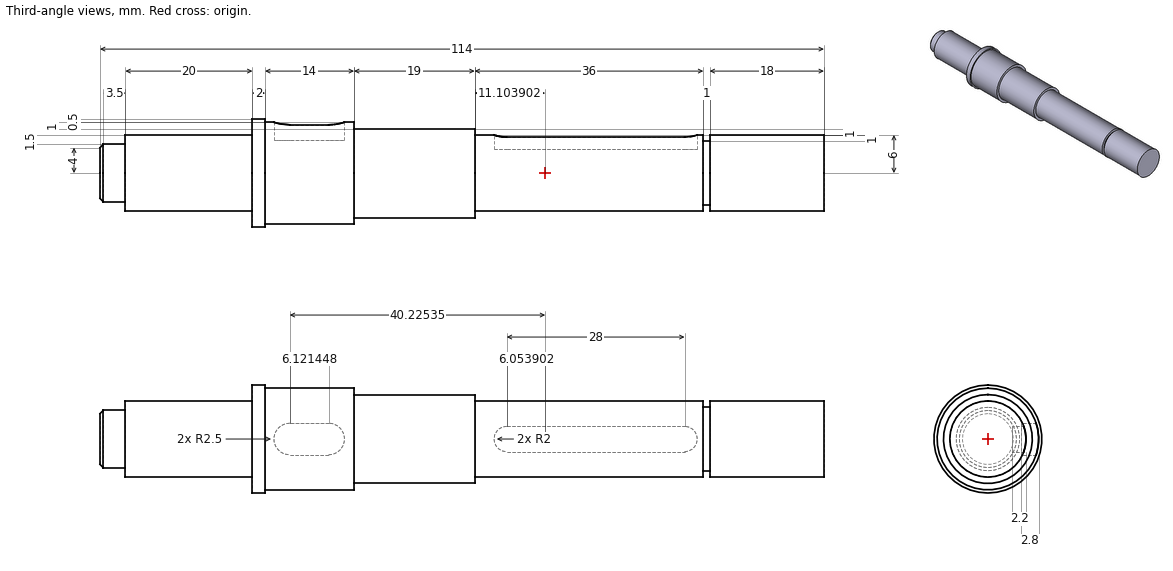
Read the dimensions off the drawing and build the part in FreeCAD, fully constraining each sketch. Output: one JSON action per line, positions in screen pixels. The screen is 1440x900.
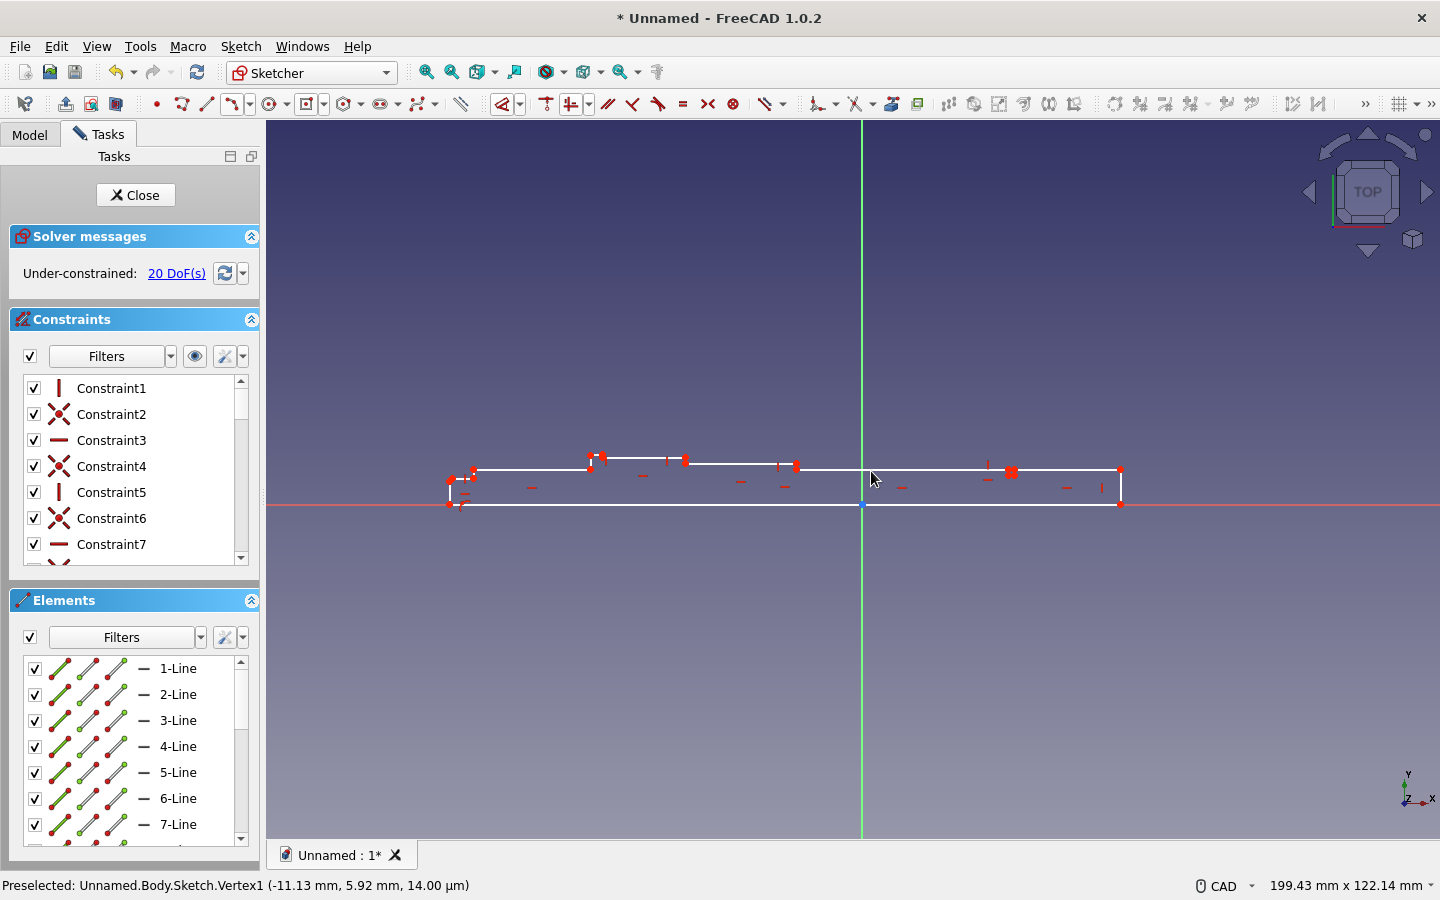
{"action": "scroll", "coordinate": [599, 455], "scroll_direction": "up", "scroll_amount": 7}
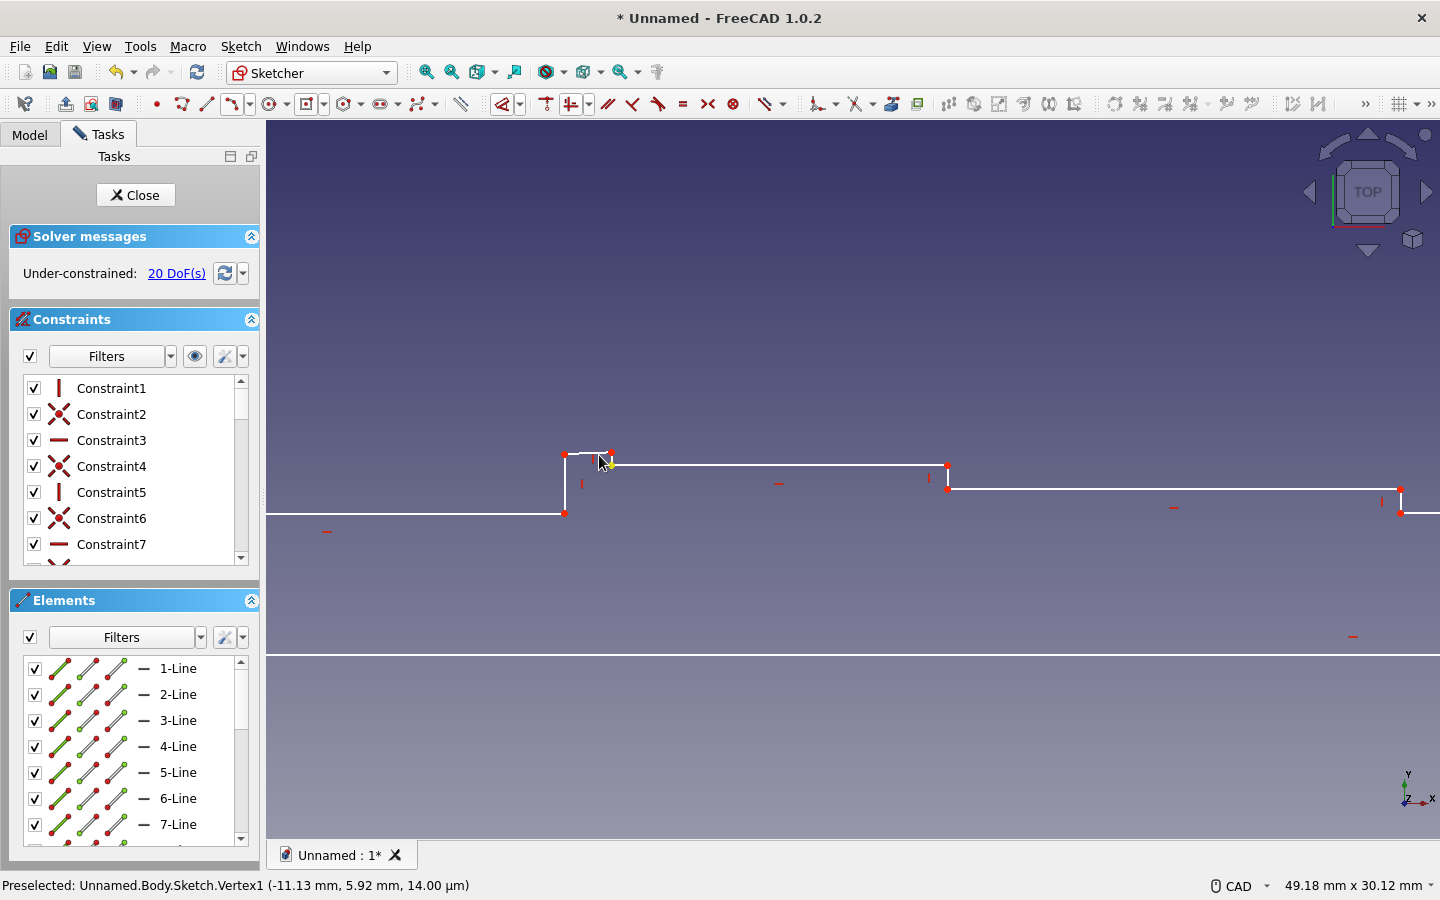
{"action": "left_click", "coordinate": [579, 453]}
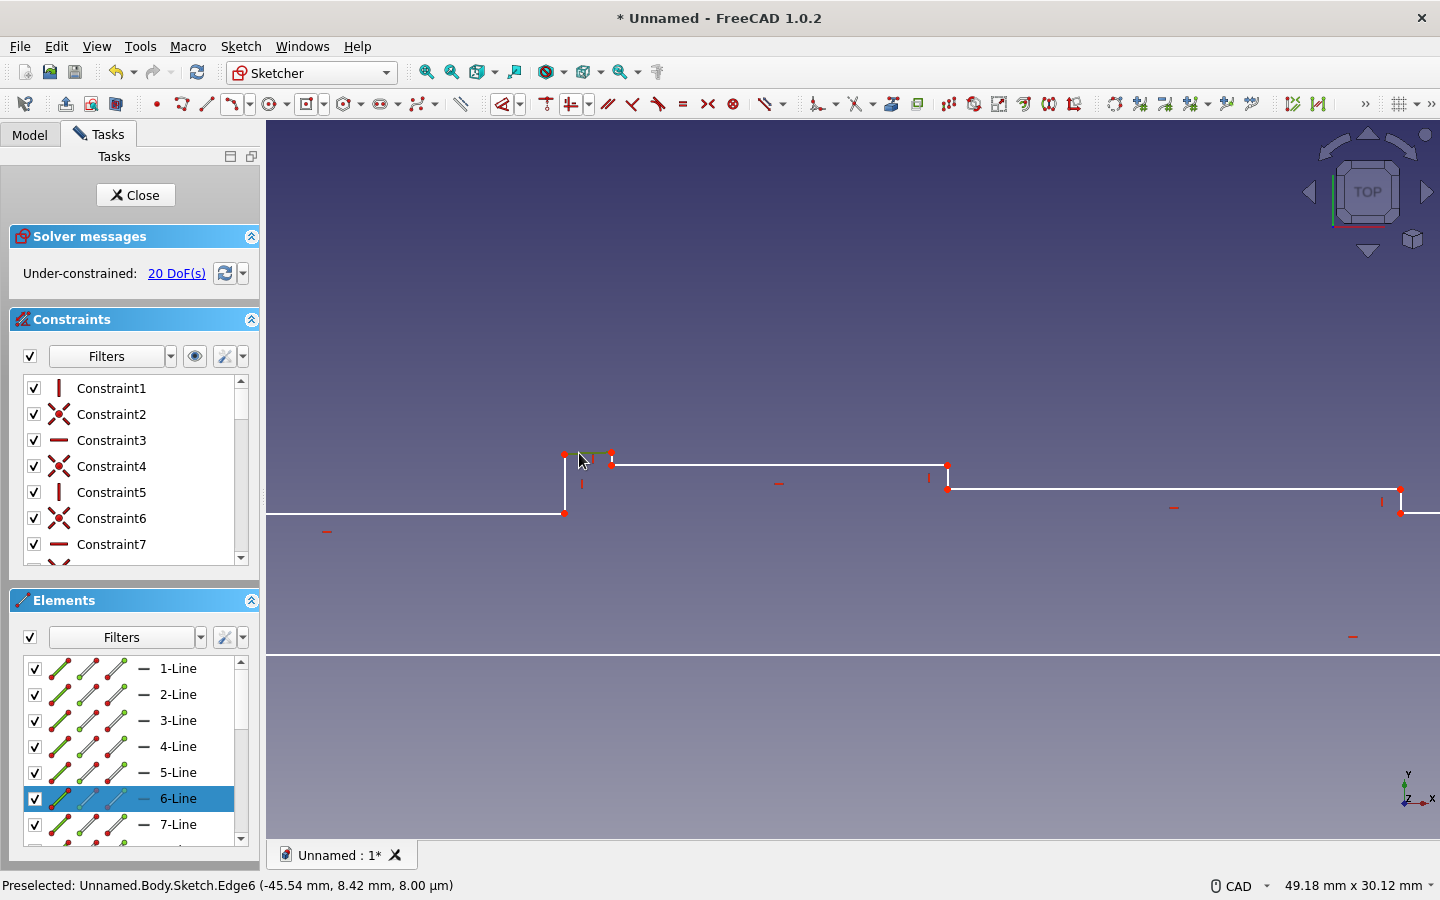
{"action": "key", "text": "h"}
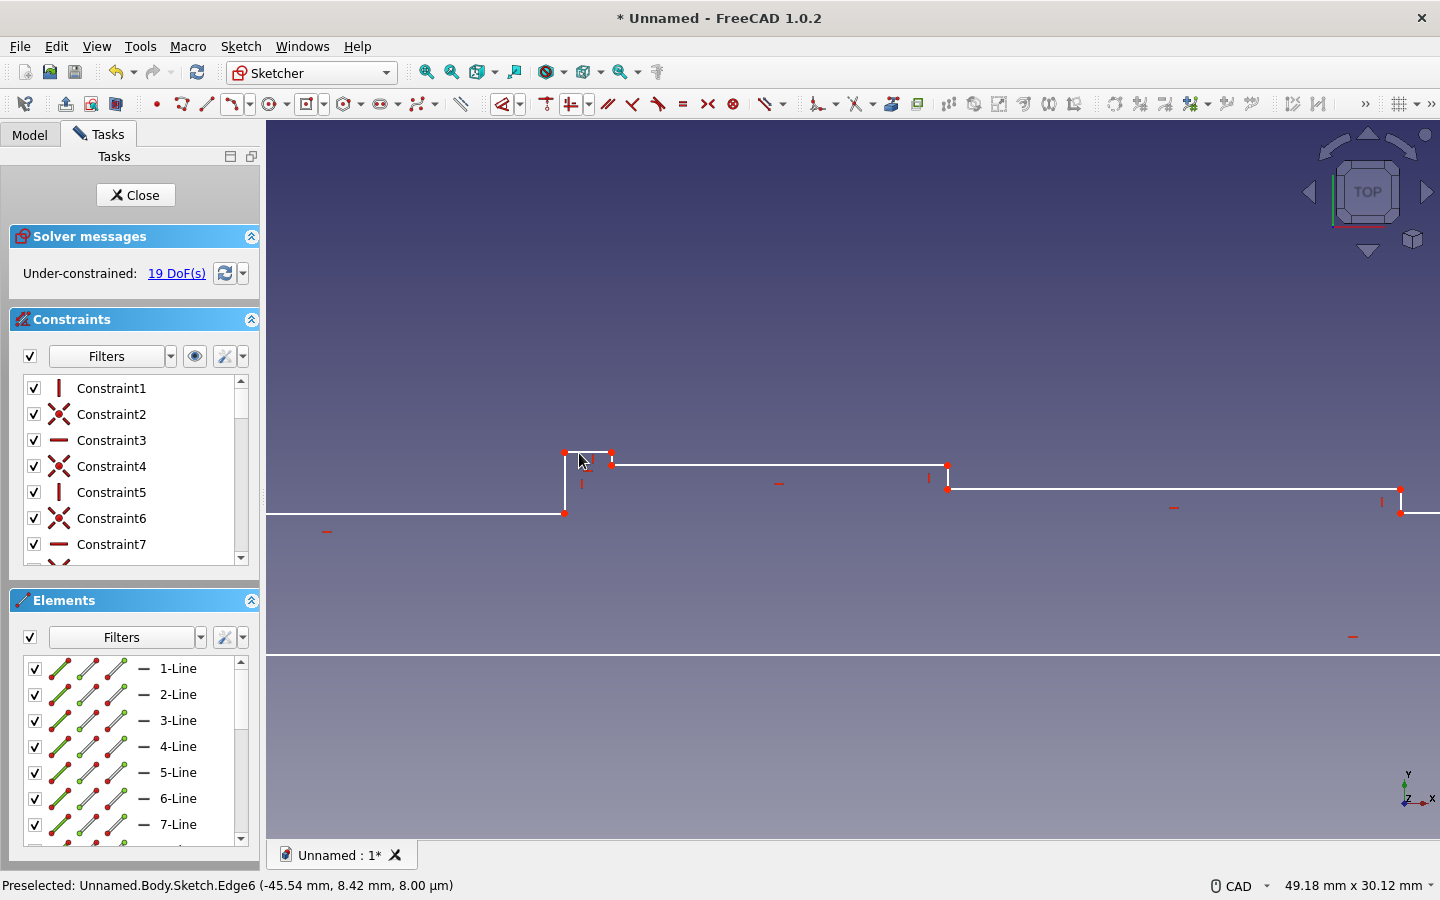
{"action": "scroll", "coordinate": [598, 455], "scroll_direction": "down", "scroll_amount": 7}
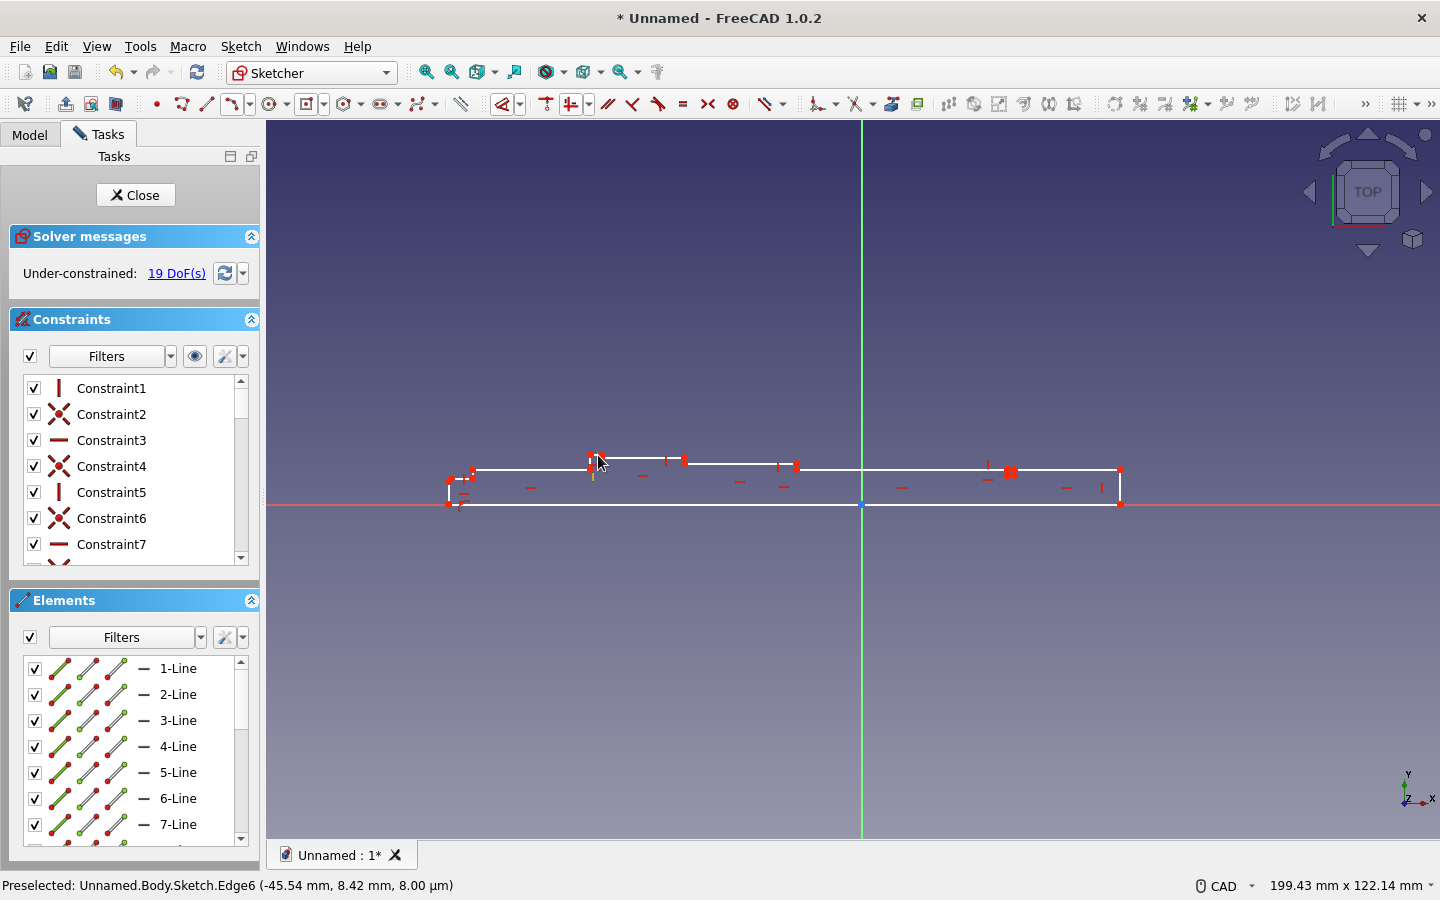
{"action": "scroll", "coordinate": [796, 467], "scroll_direction": "up", "scroll_amount": 10}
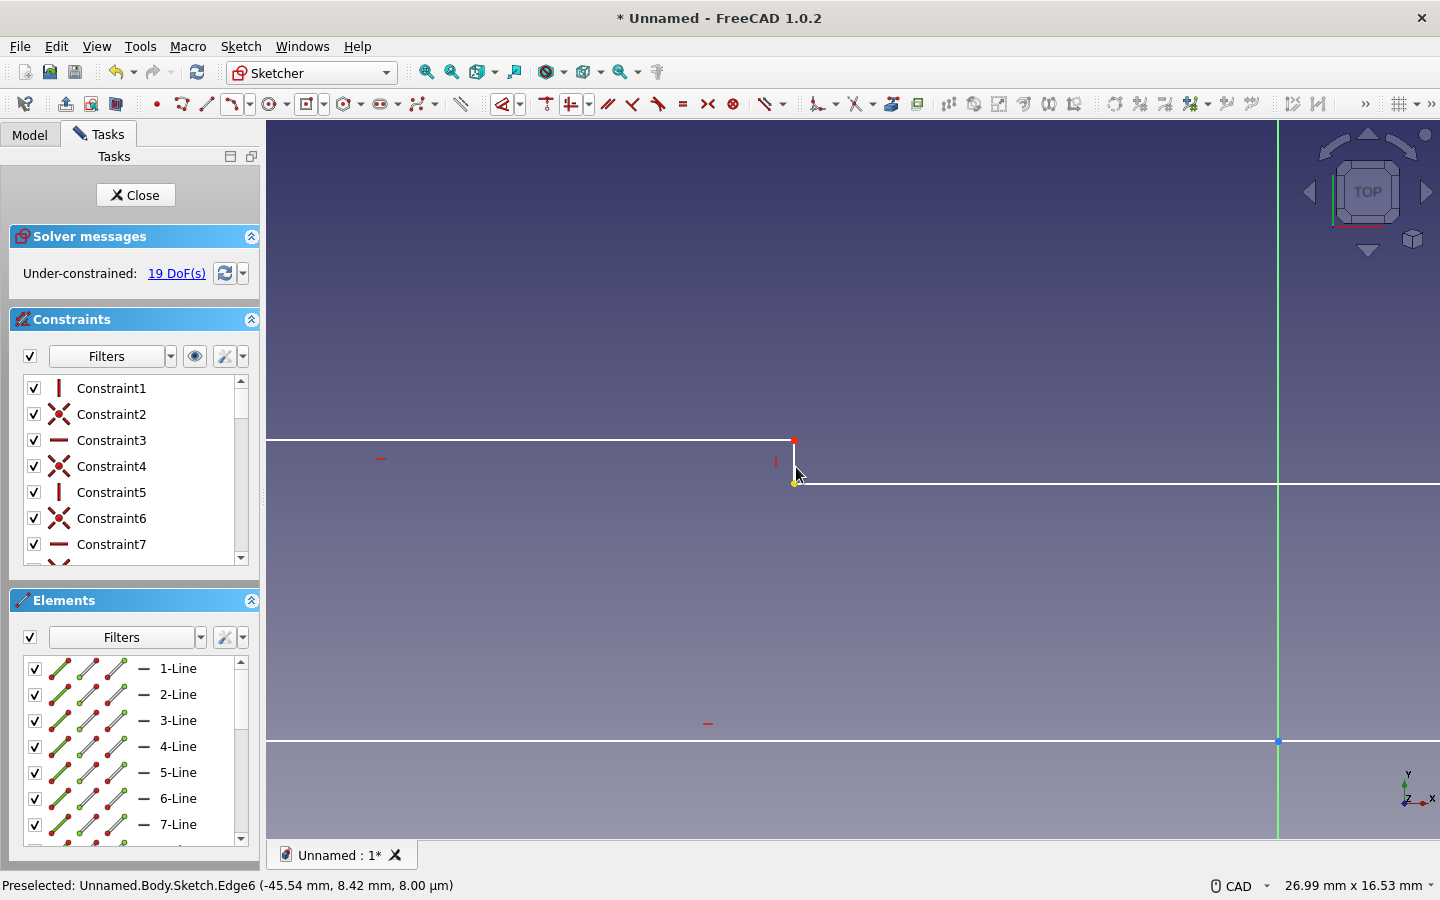
{"action": "left_click", "coordinate": [794, 466]}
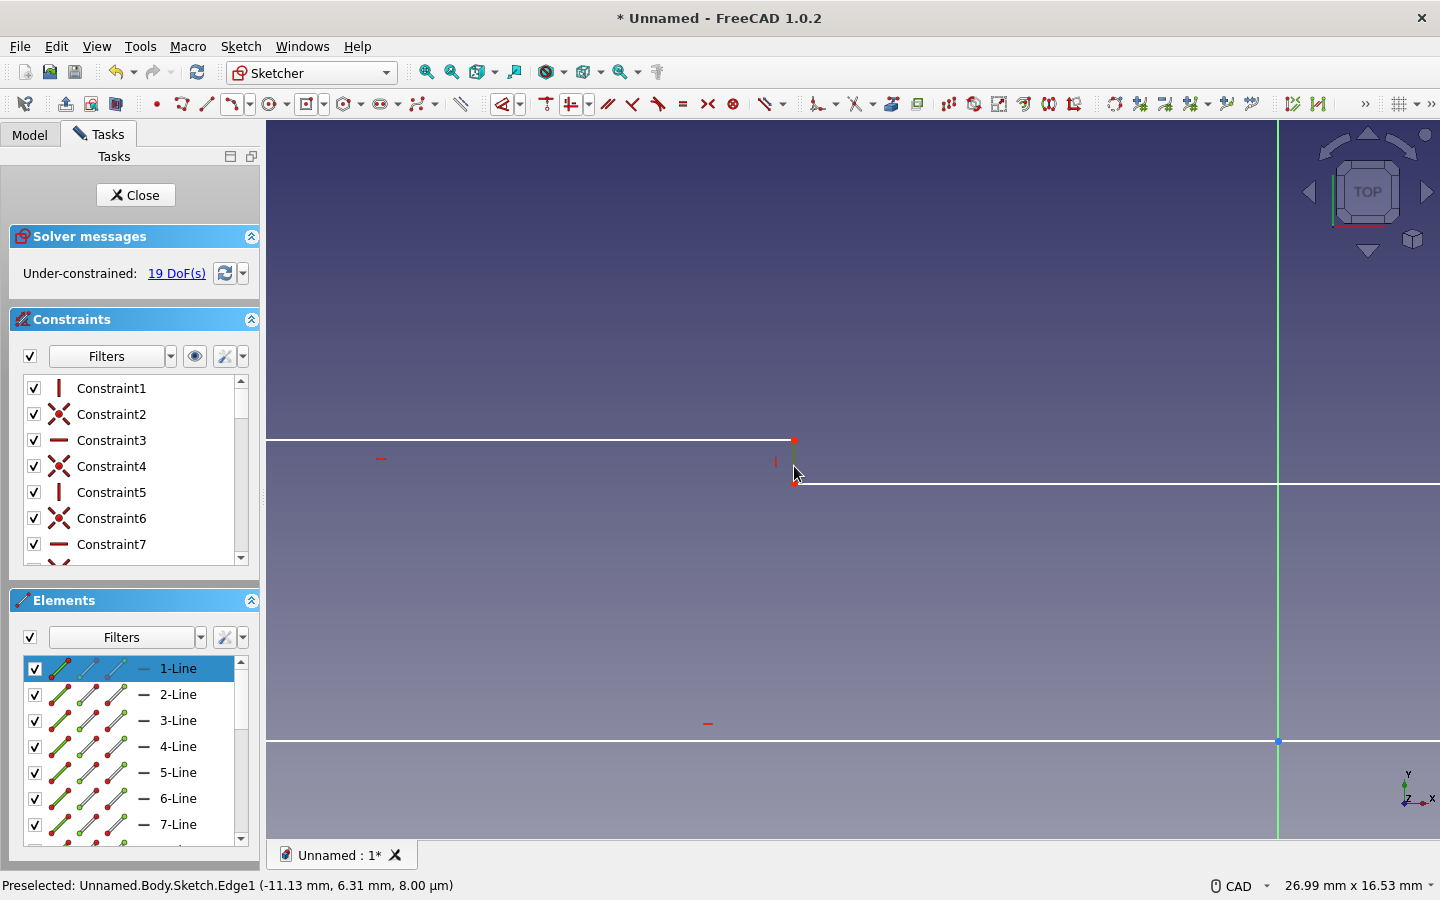
{"action": "left_click", "coordinate": [520, 104]}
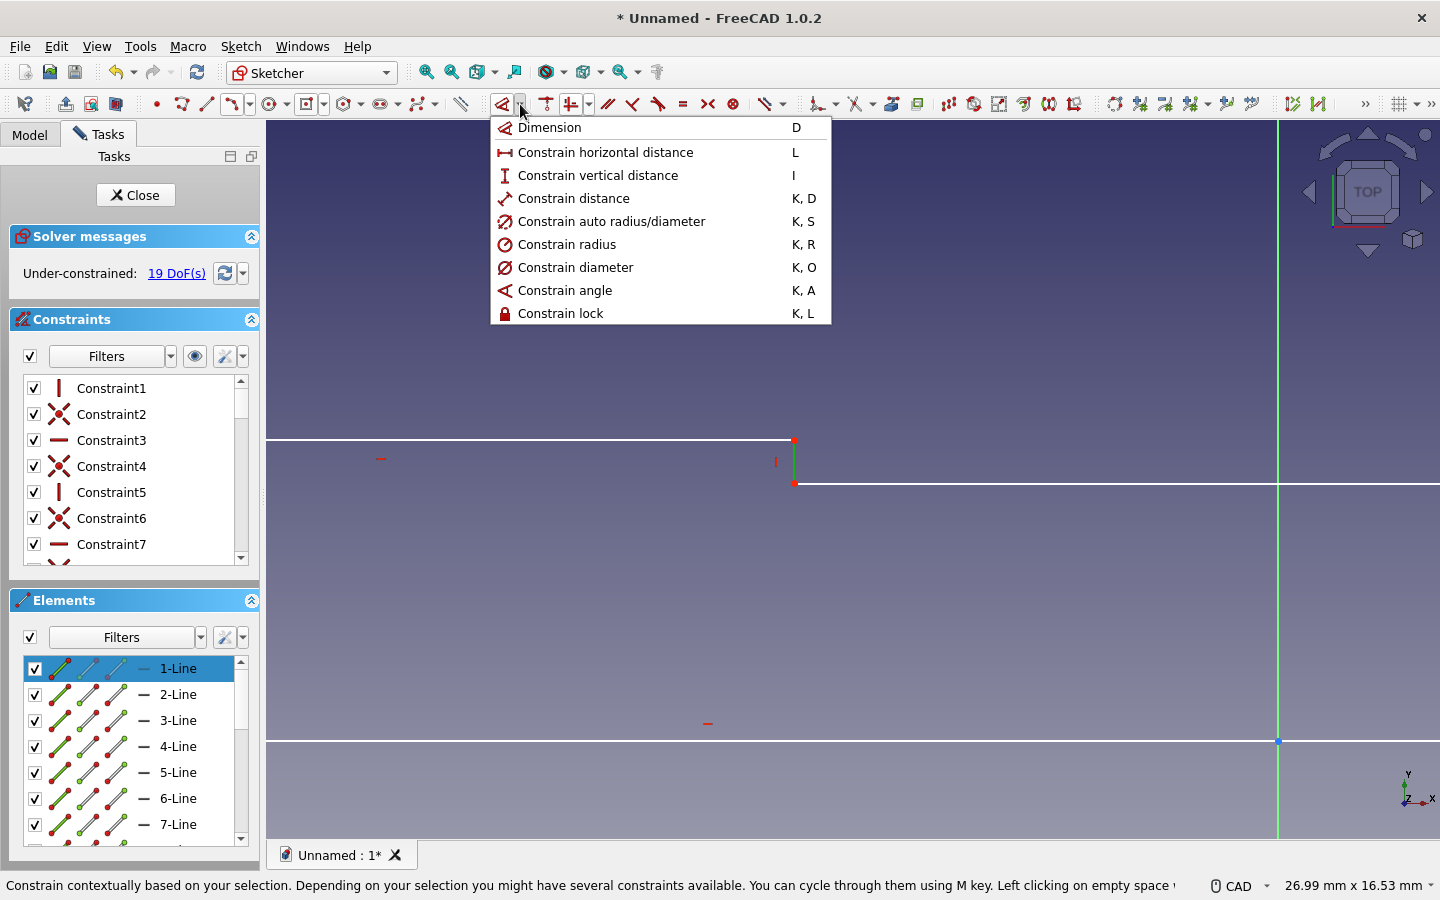
{"action": "left_click", "coordinate": [661, 176]}